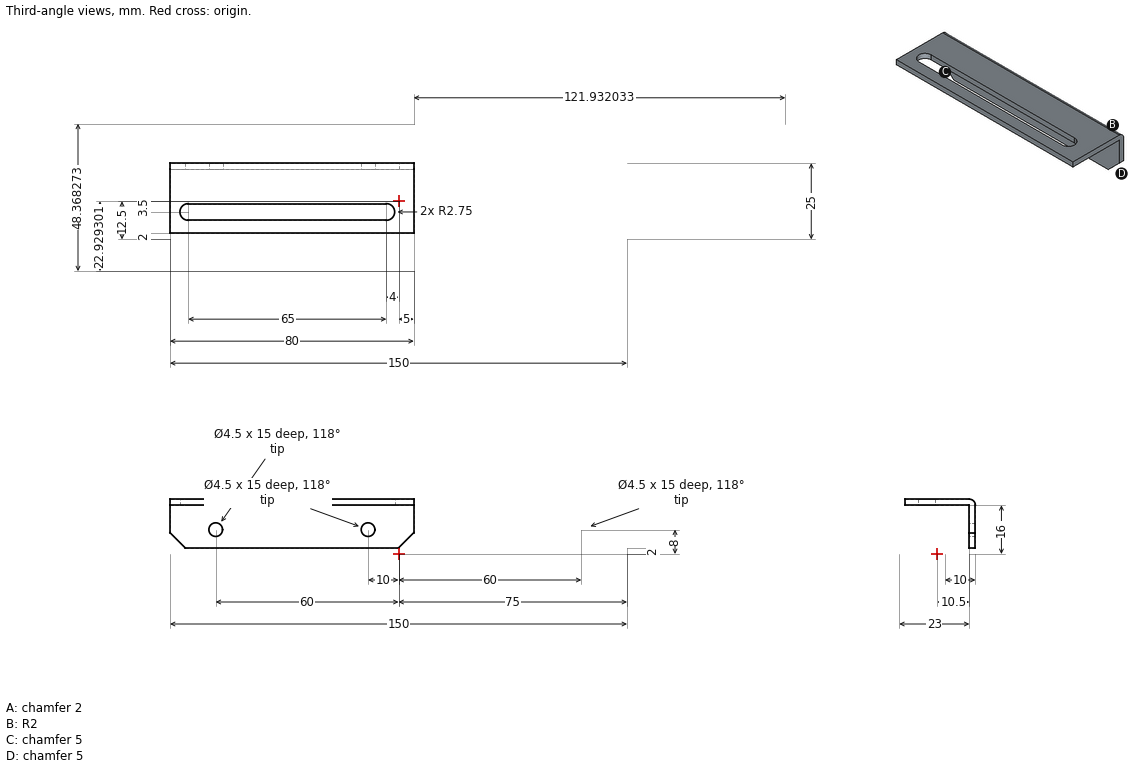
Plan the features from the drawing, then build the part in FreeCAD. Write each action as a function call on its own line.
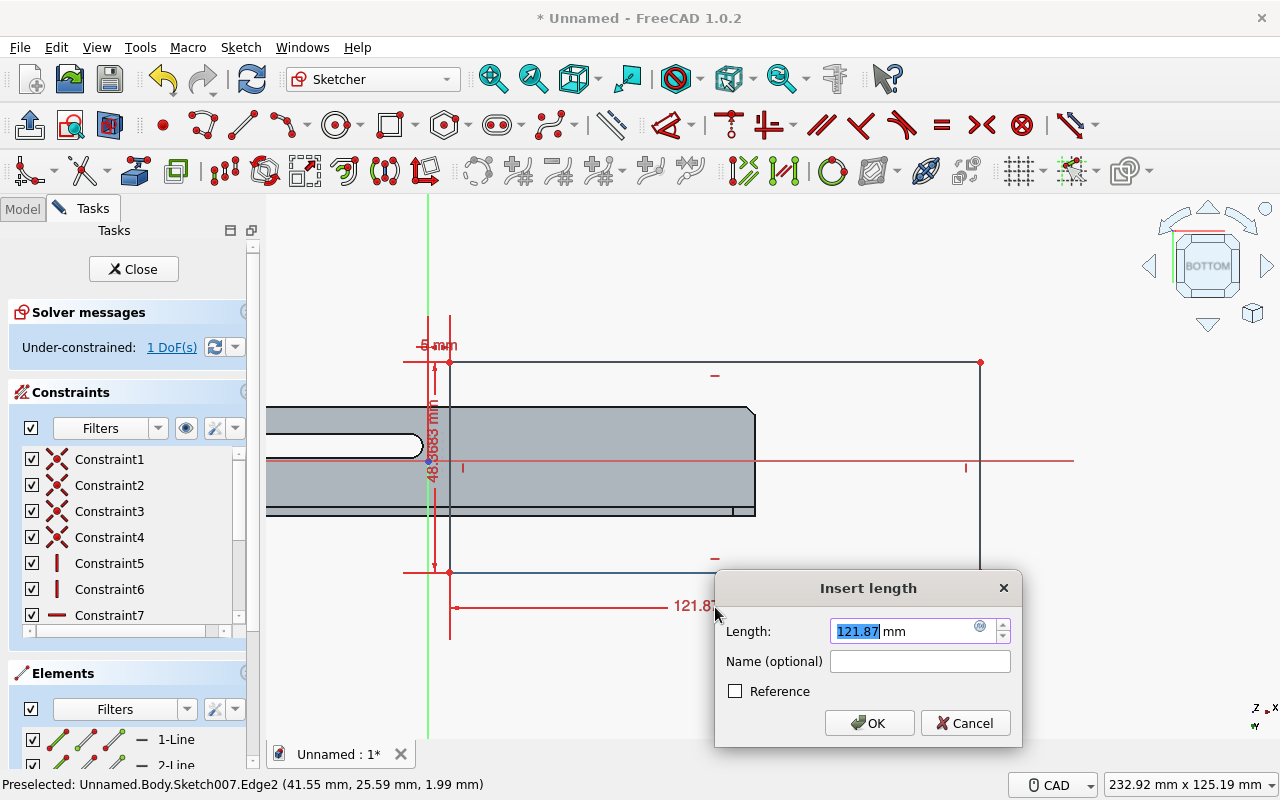
text(121.932033)
key(Return)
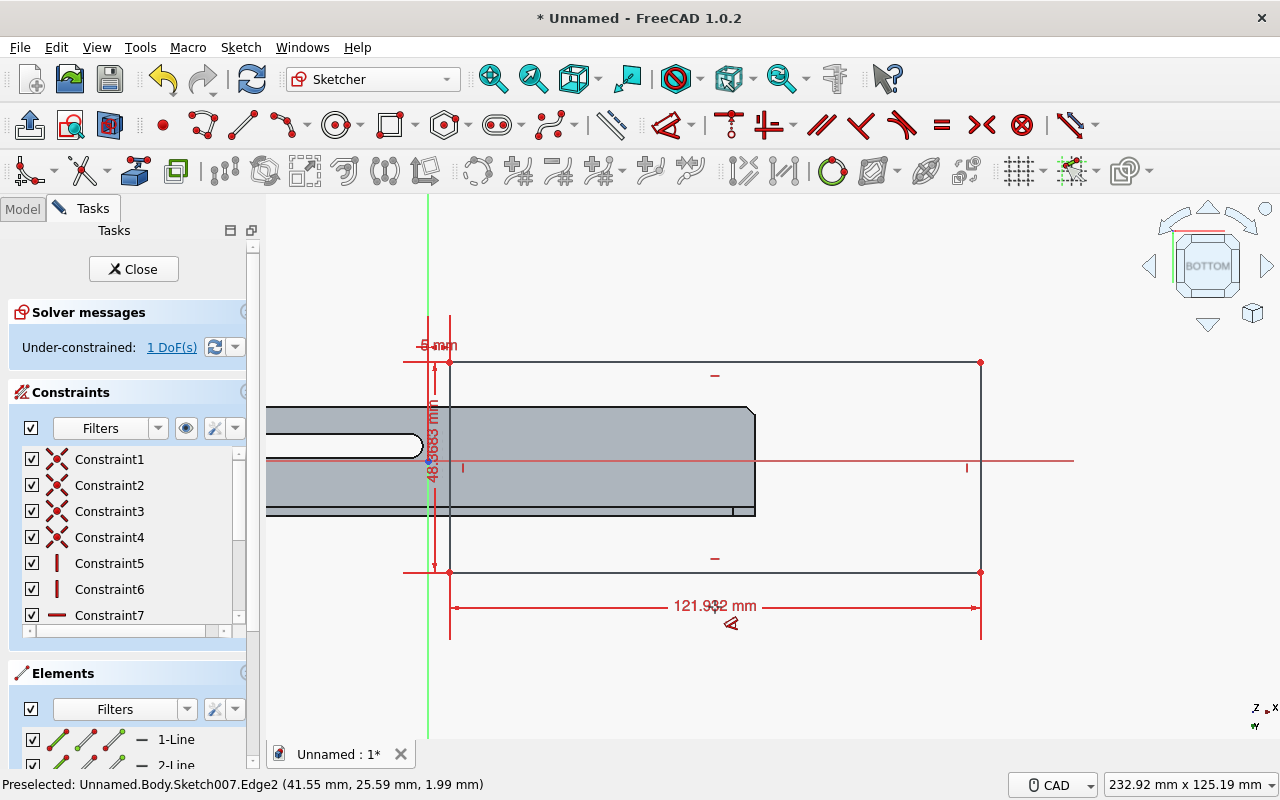
click(450, 362)
click(394, 412)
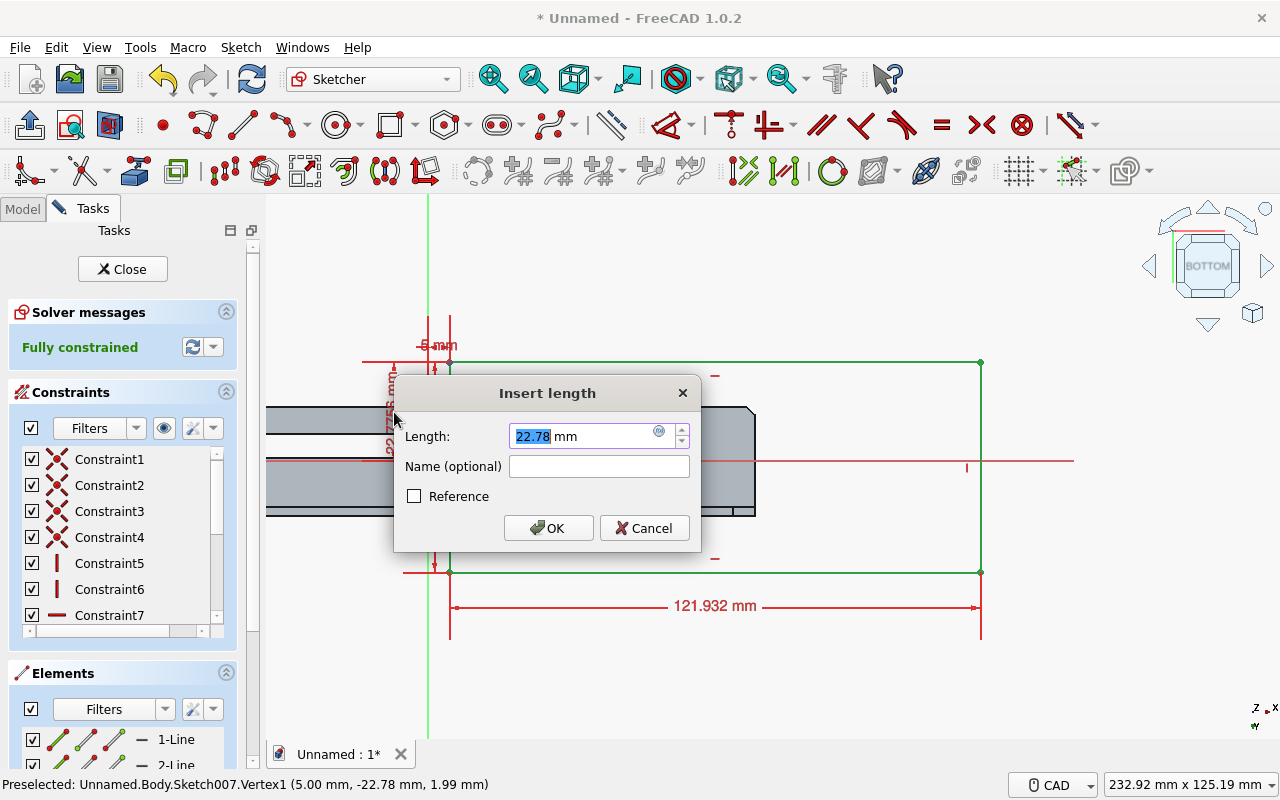
text(22.929301)
key(Return)
key(Escape)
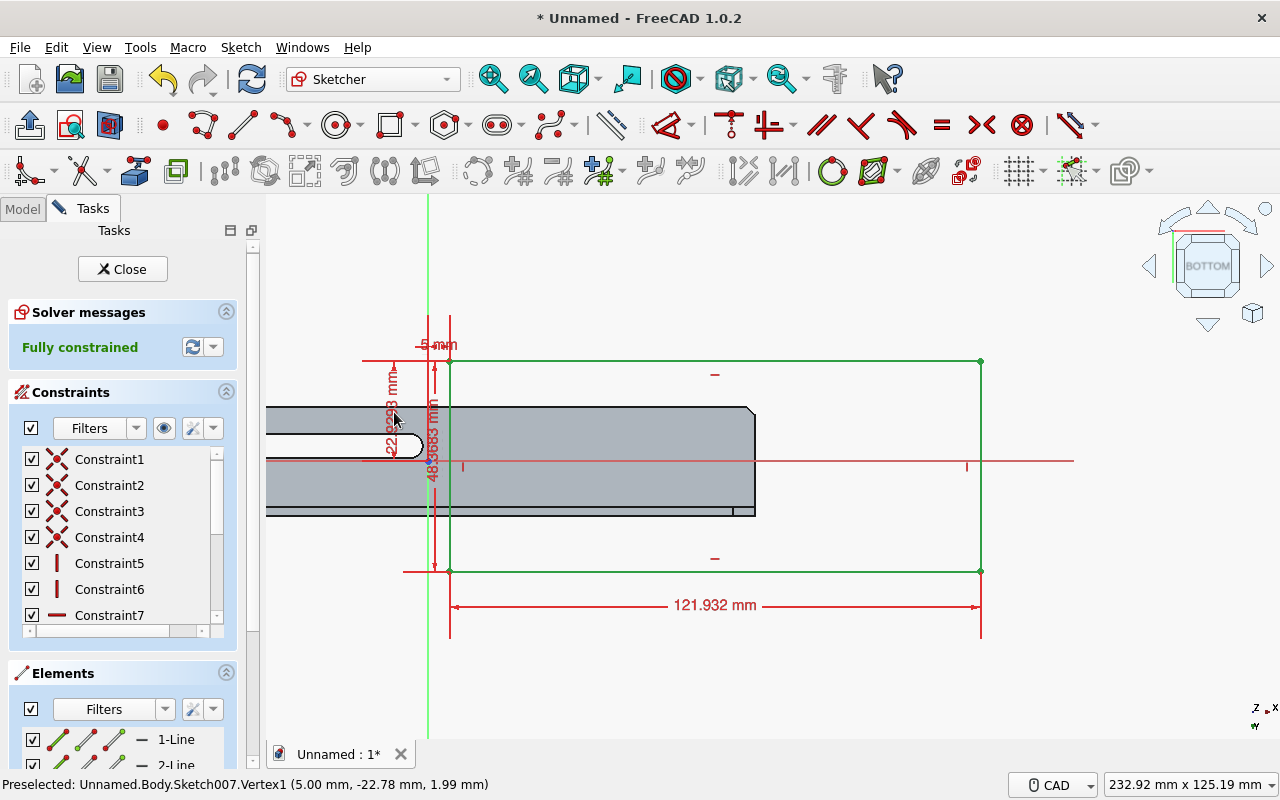
click(123, 269)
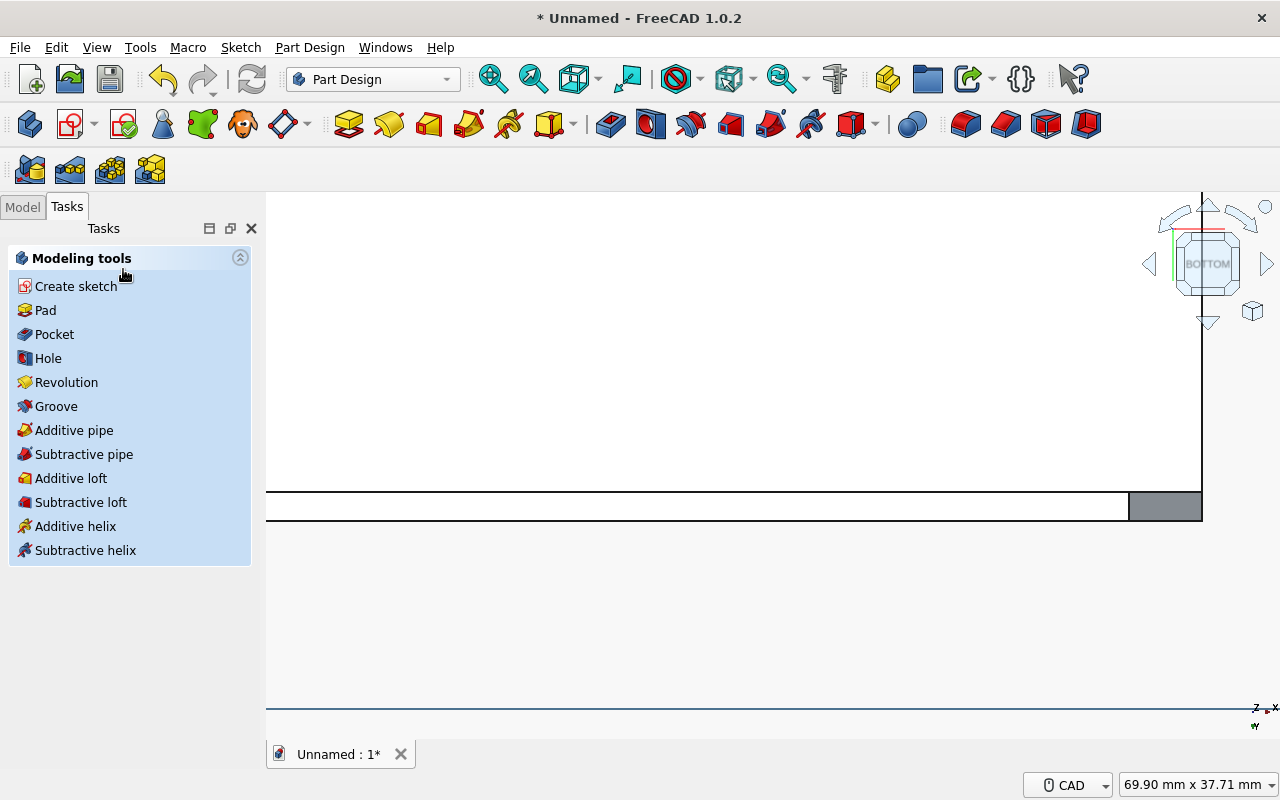
click(612, 124)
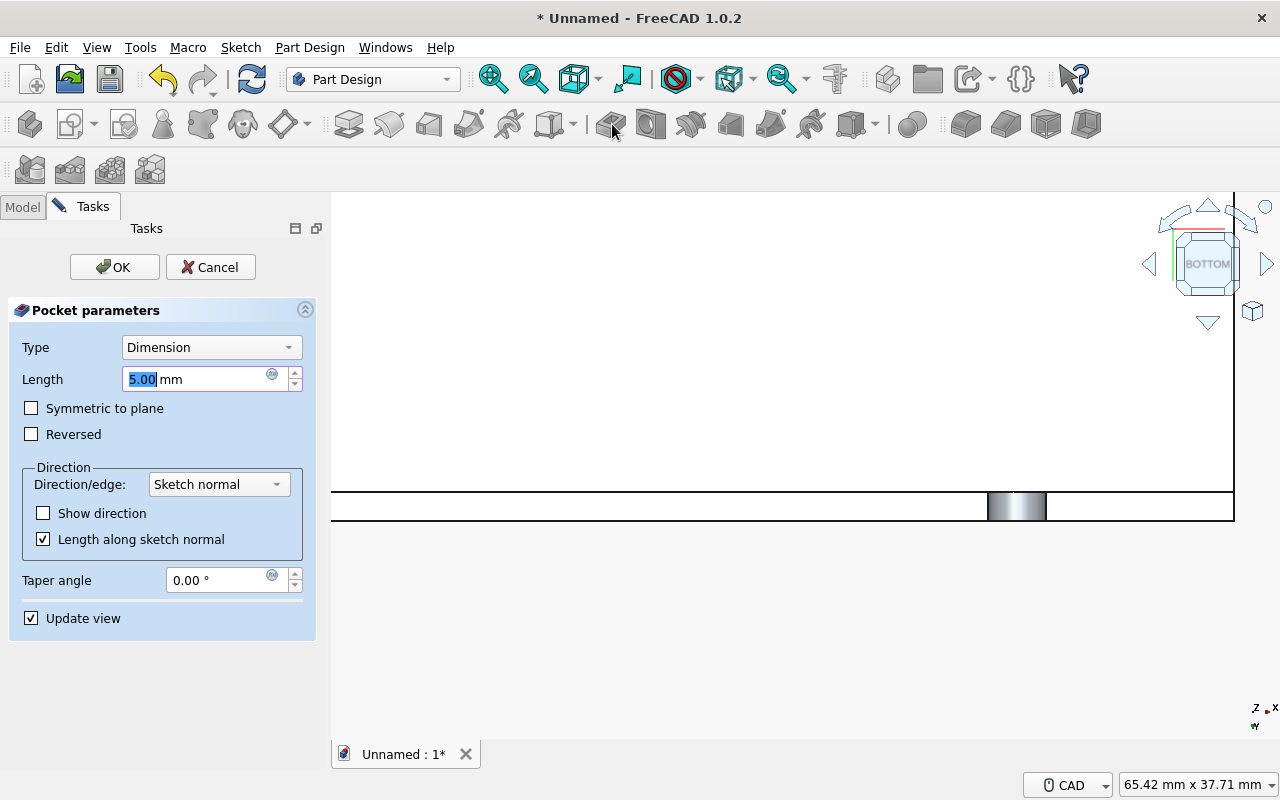
click(212, 348)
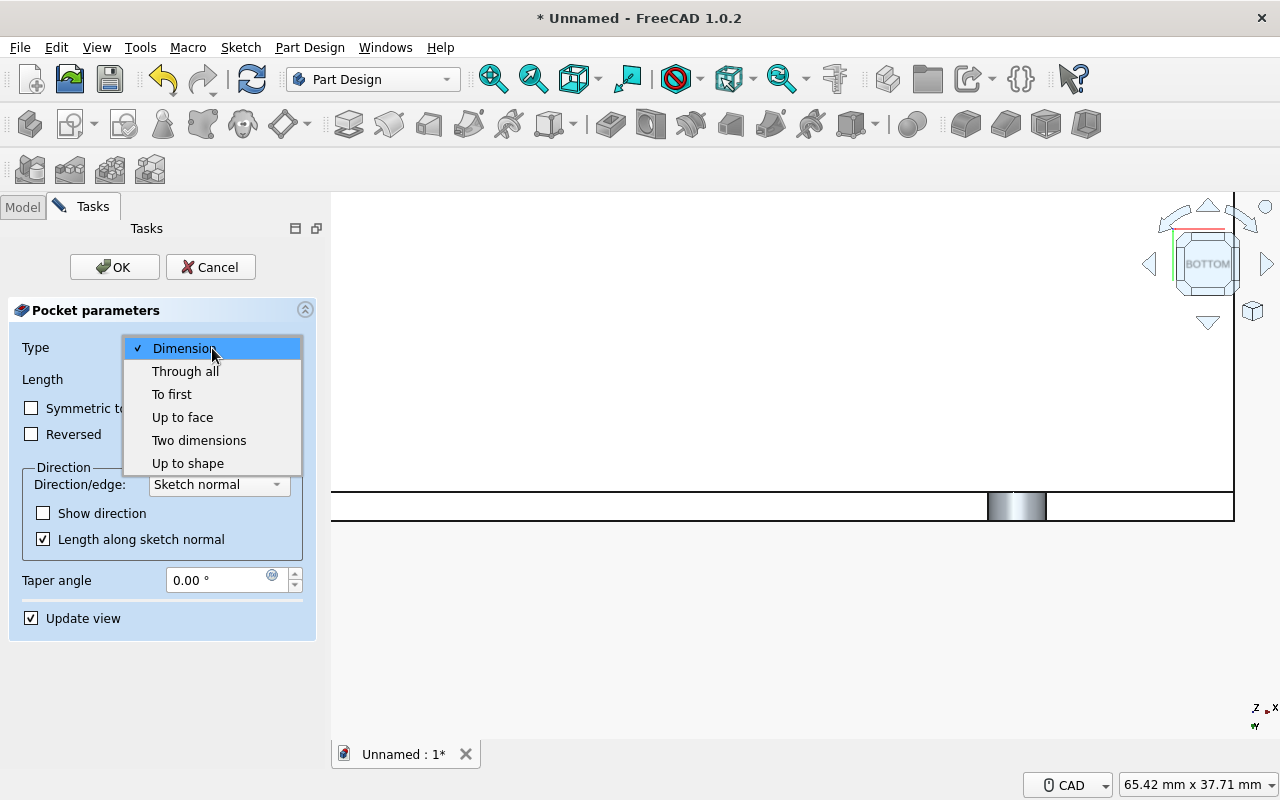
click(212, 372)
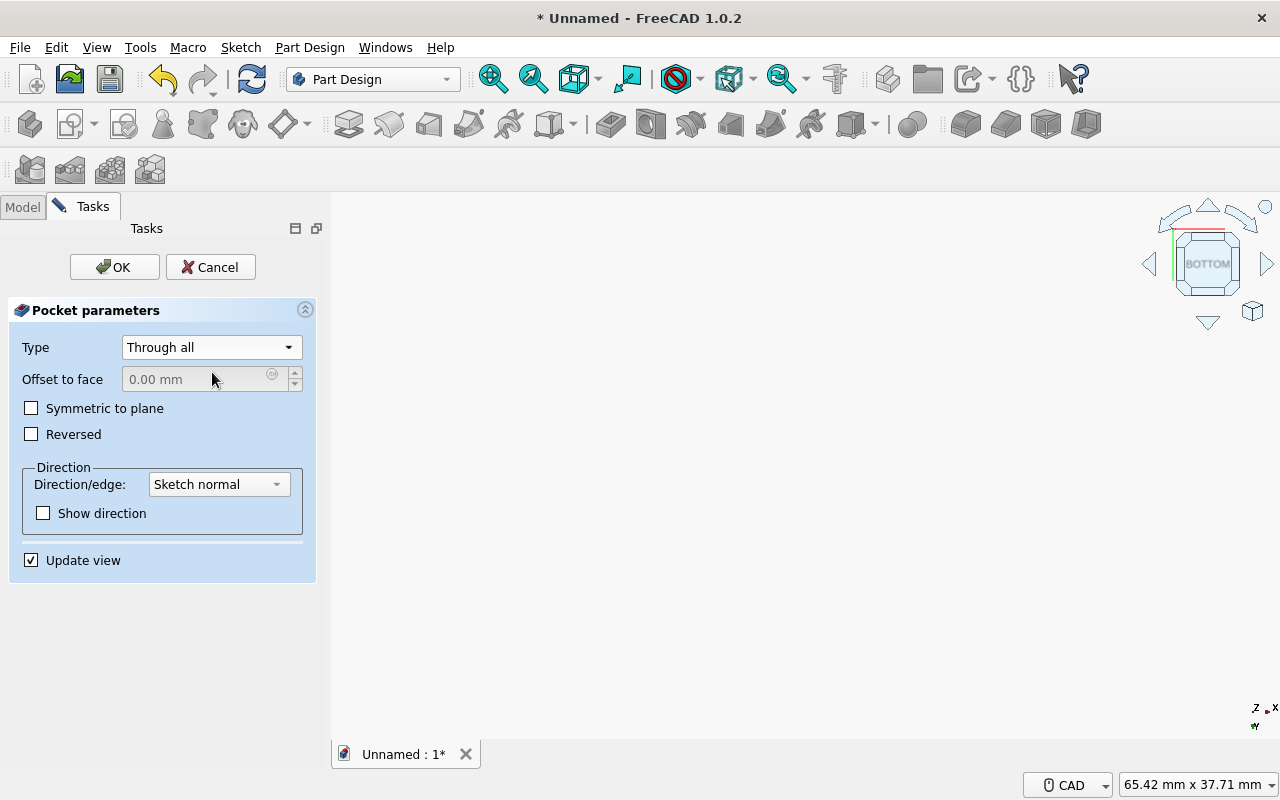
click(115, 267)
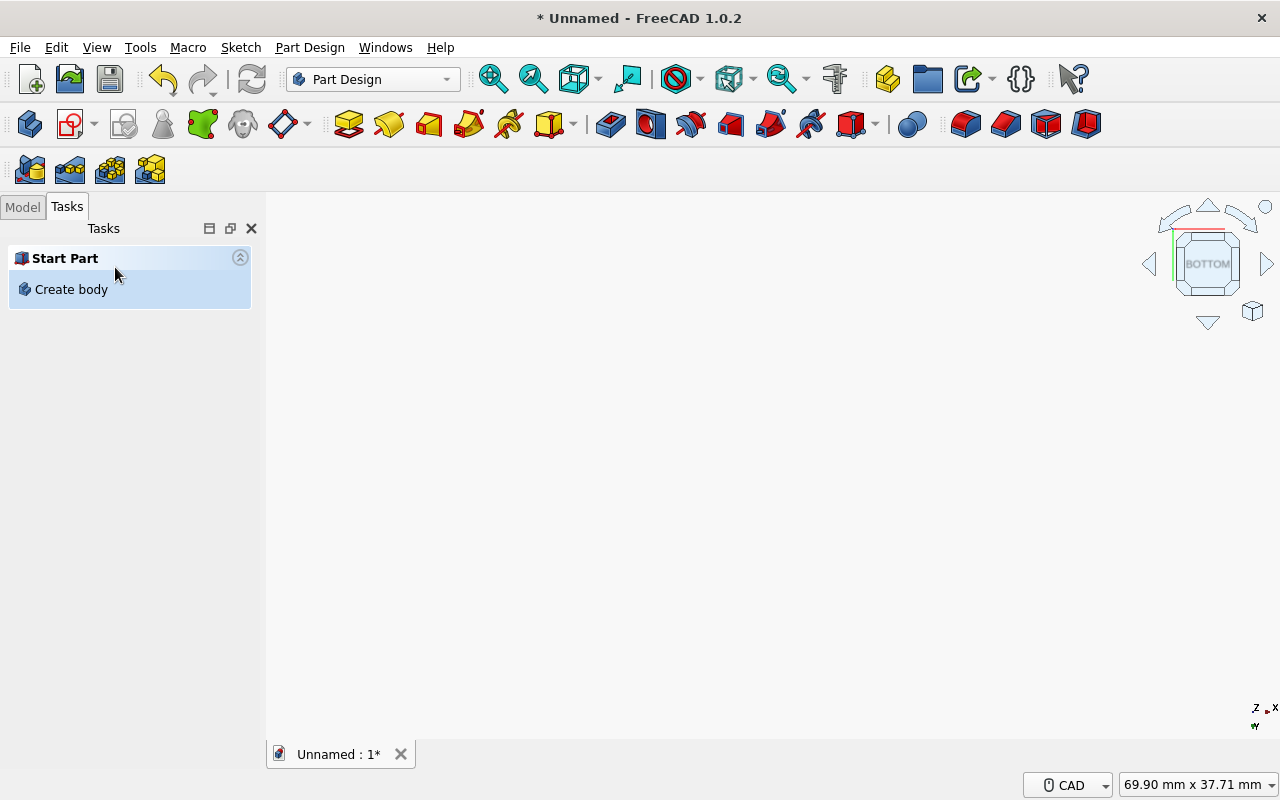
click(494, 80)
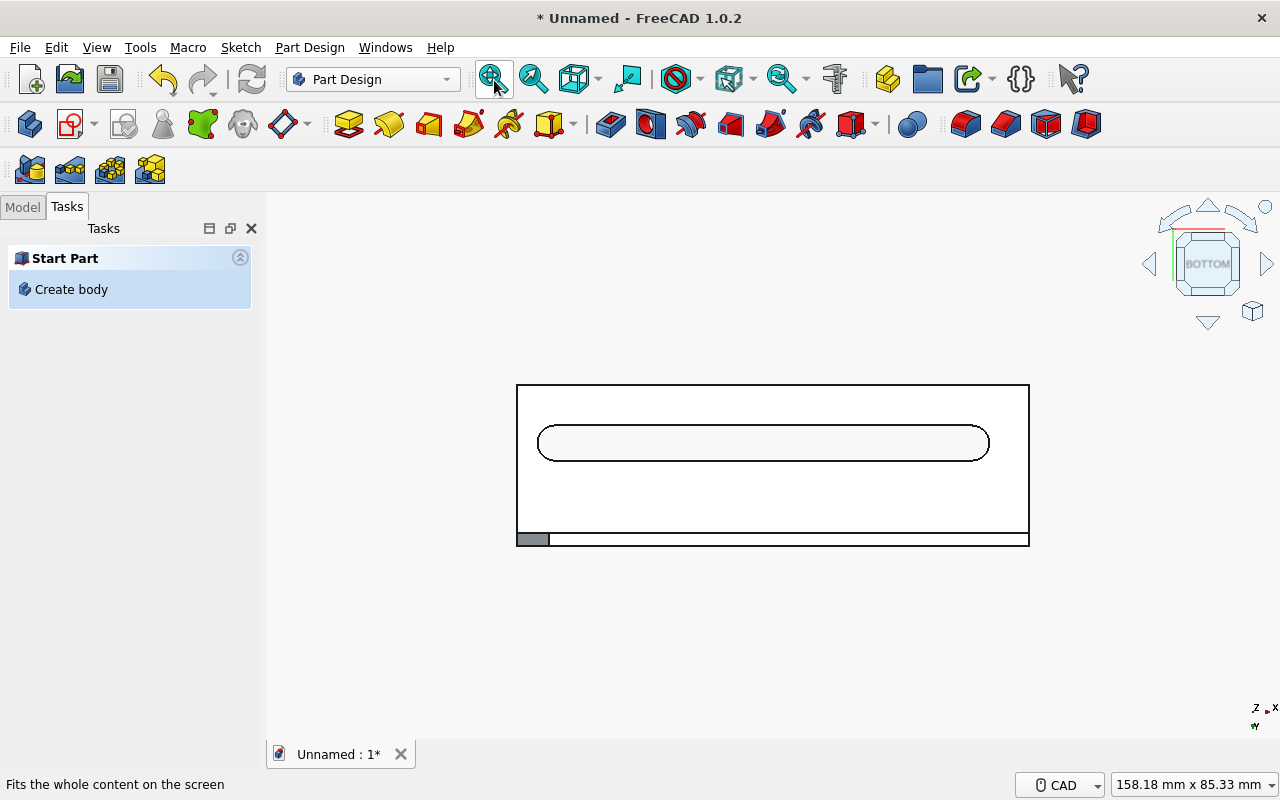
click(1029, 538)